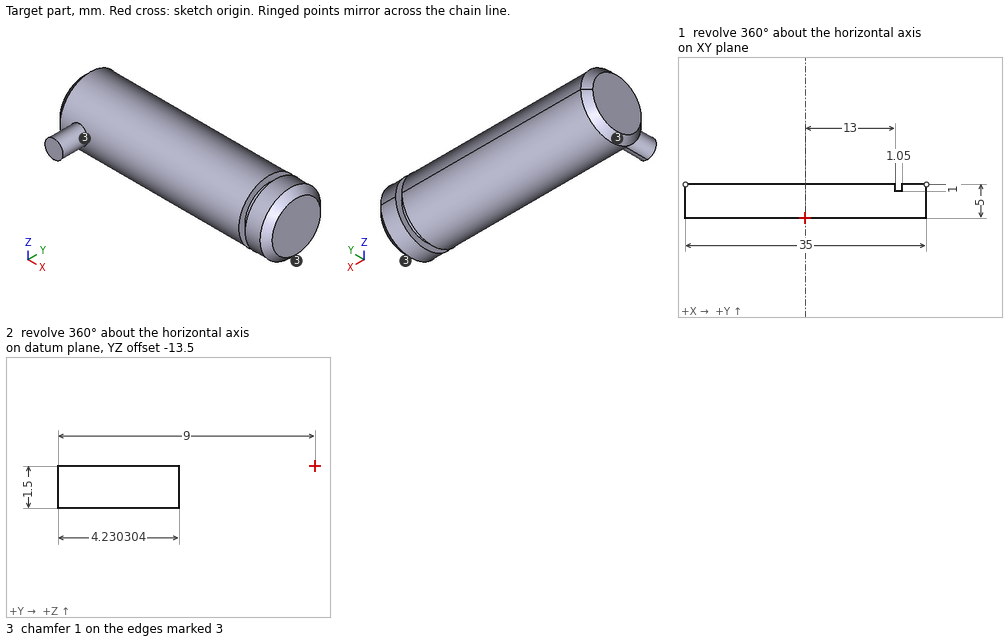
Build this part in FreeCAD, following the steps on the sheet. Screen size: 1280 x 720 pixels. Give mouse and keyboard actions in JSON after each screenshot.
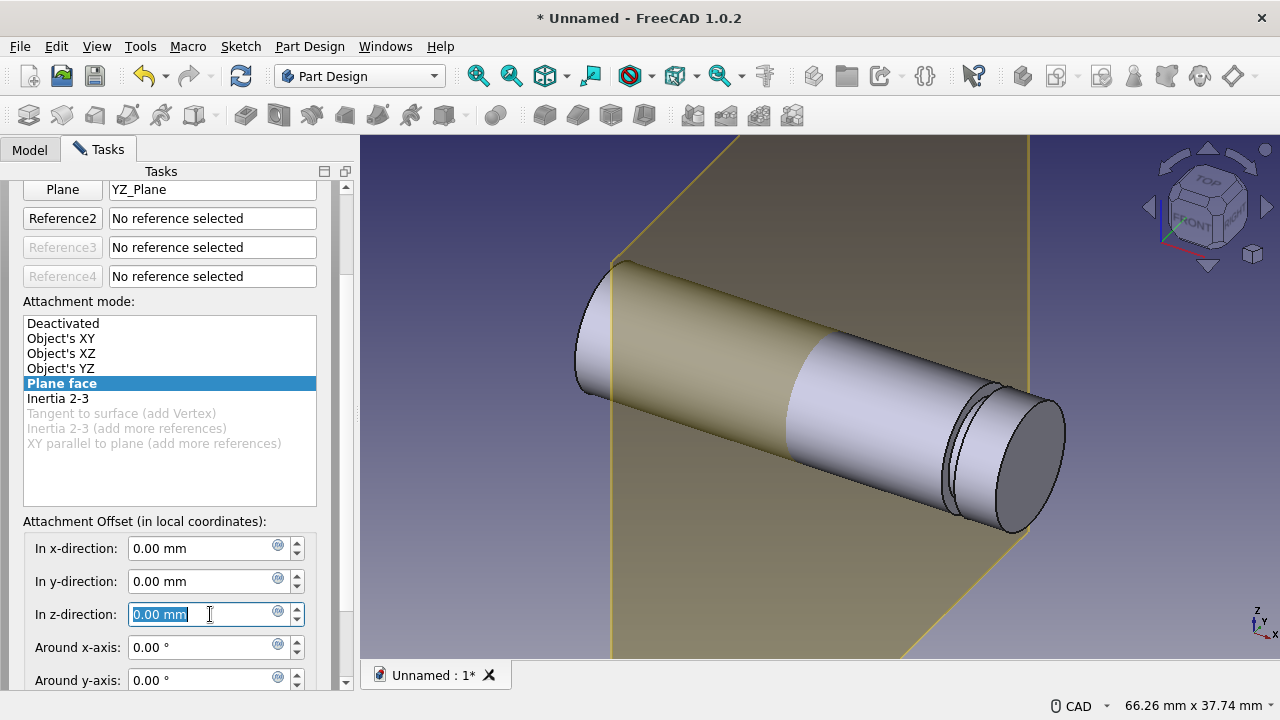
{"action": "type", "text": "-13.5"}
{"action": "key", "text": "Tab"}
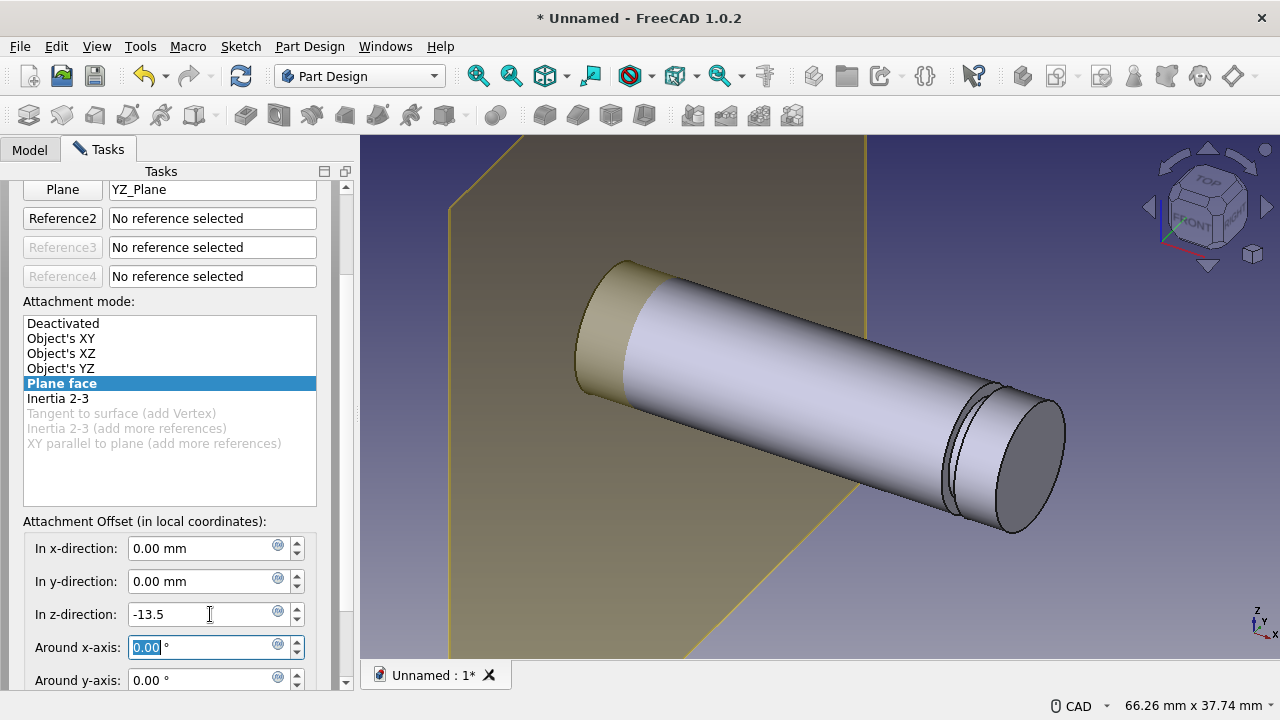
{"action": "scroll", "coordinate": [346, 436], "scroll_direction": "up", "scroll_amount": 3}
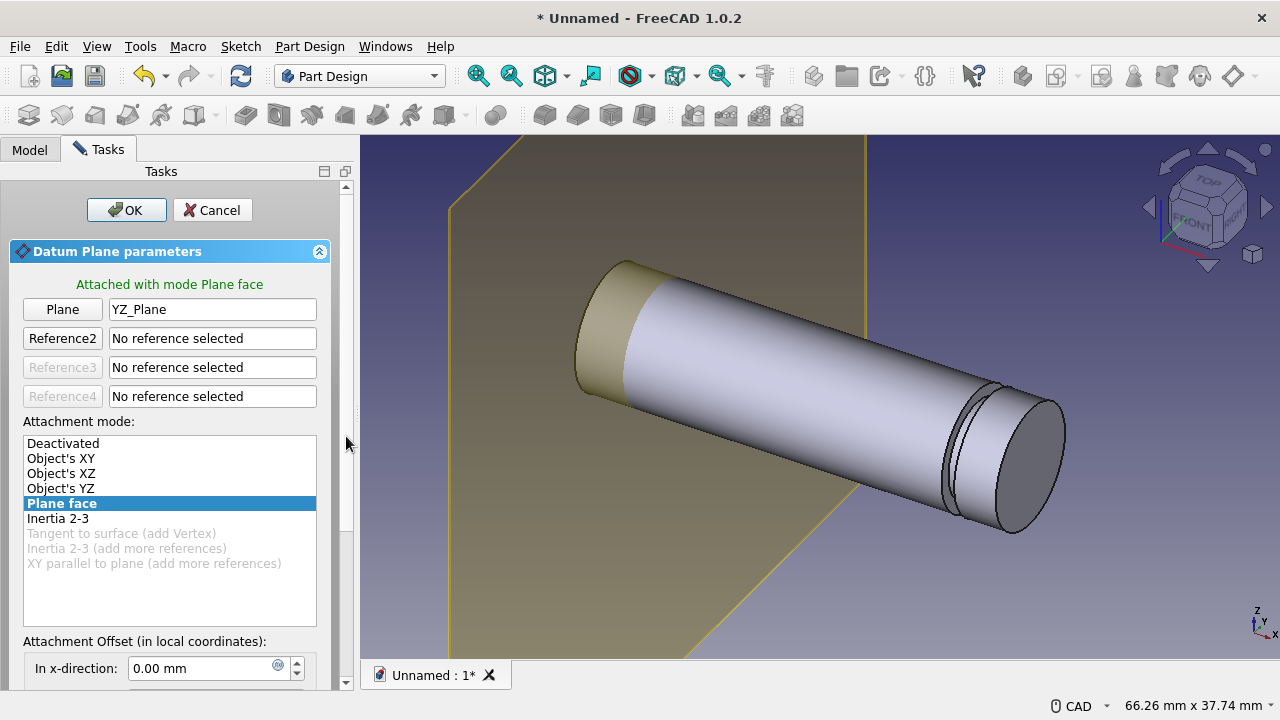
{"action": "left_click", "coordinate": [127, 210]}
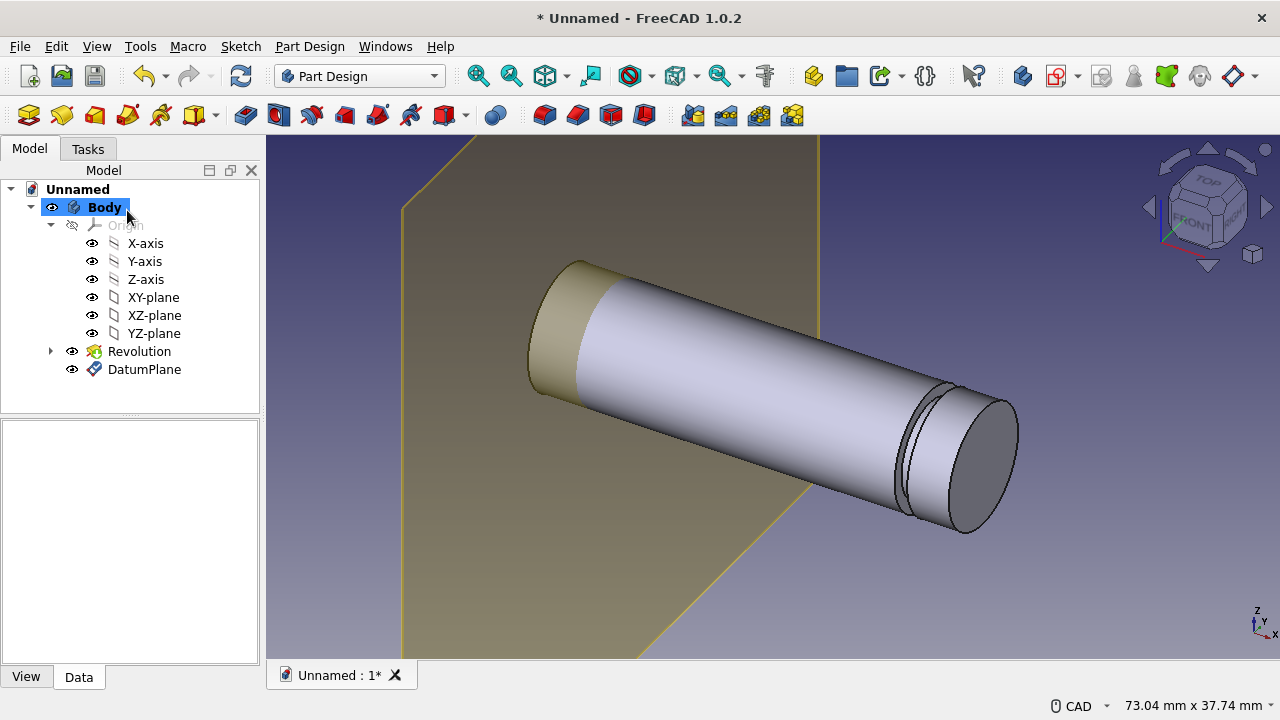
{"action": "left_click", "coordinate": [117, 369]}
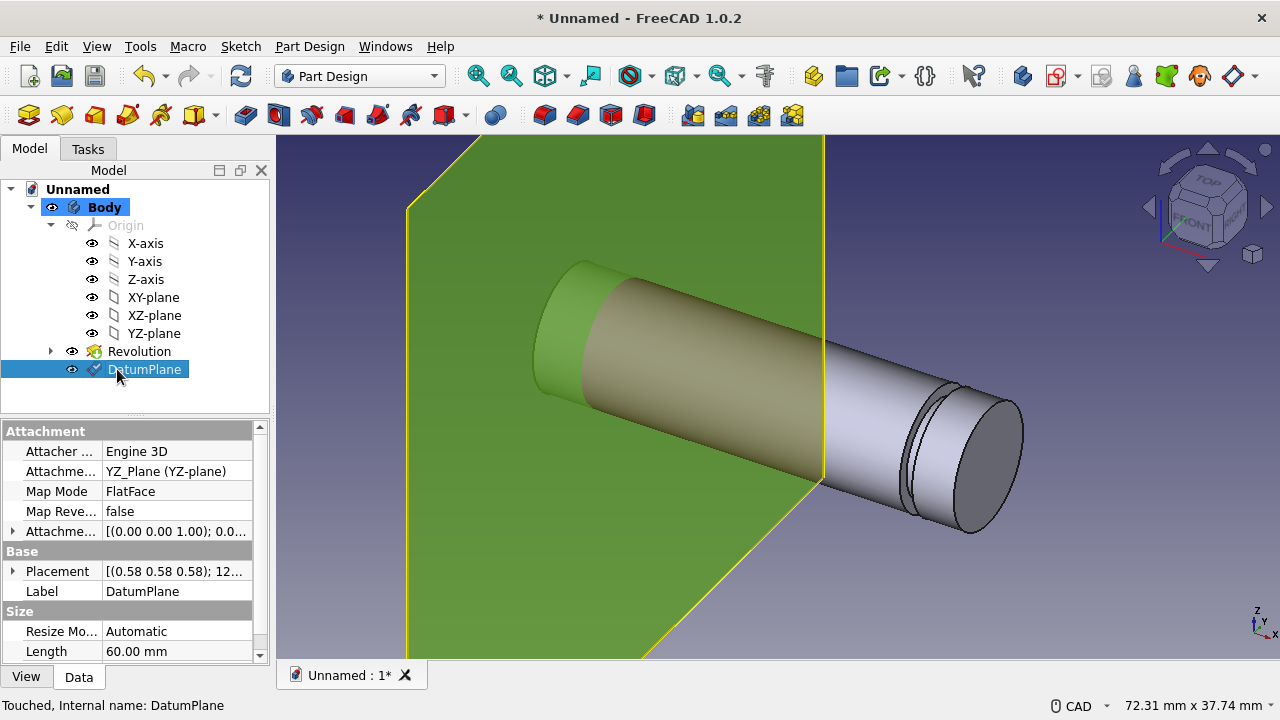
{"action": "left_click", "coordinate": [1056, 76]}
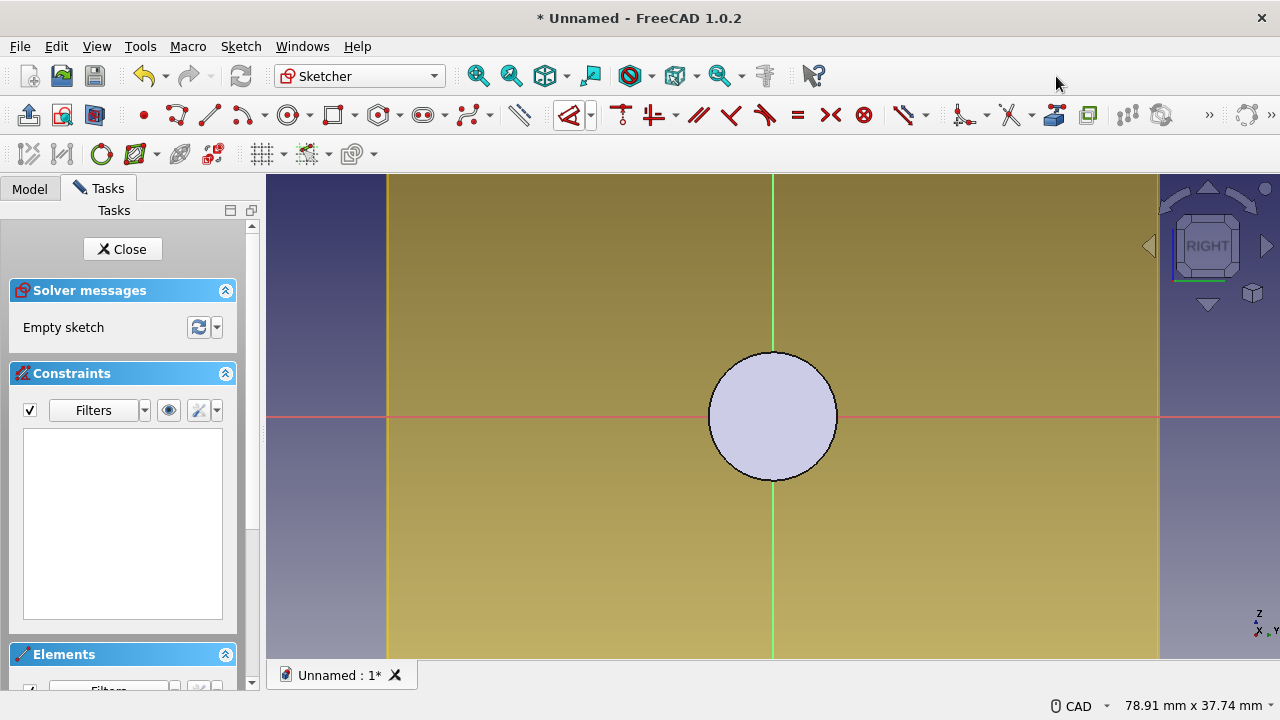
{"action": "left_click", "coordinate": [95, 116]}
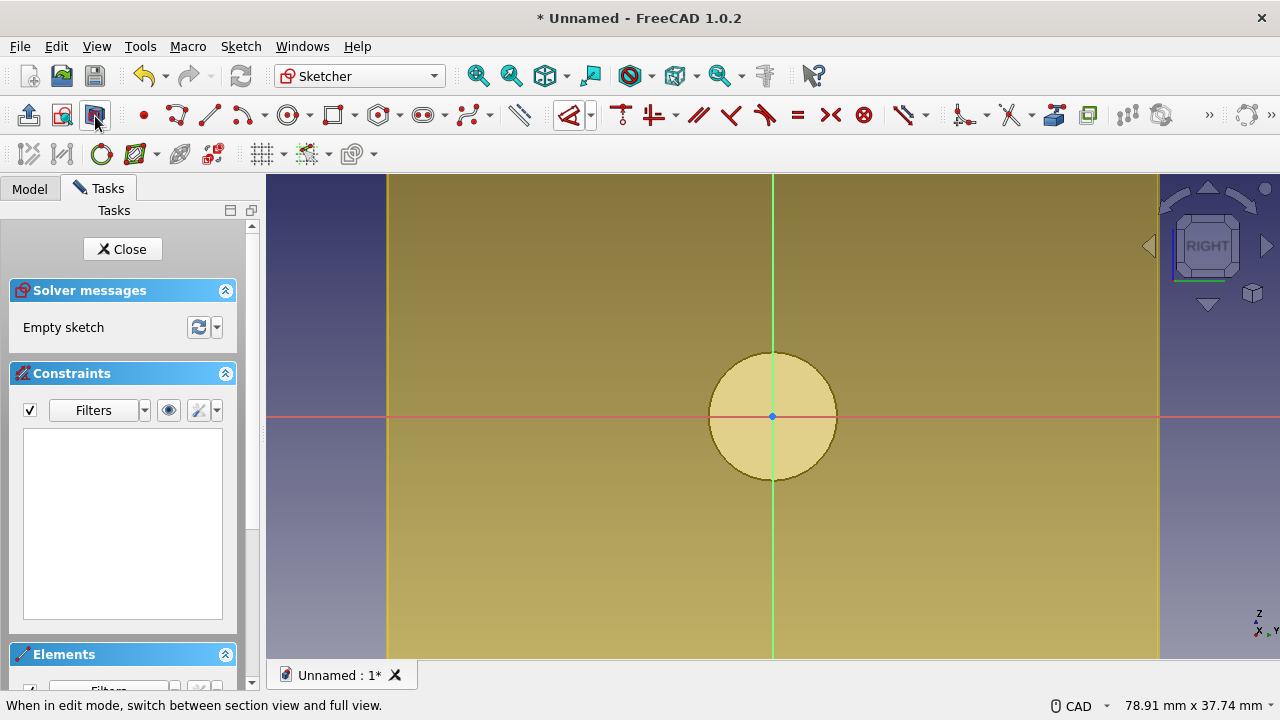
{"action": "scroll", "coordinate": [718, 429], "scroll_direction": "up", "scroll_amount": 8}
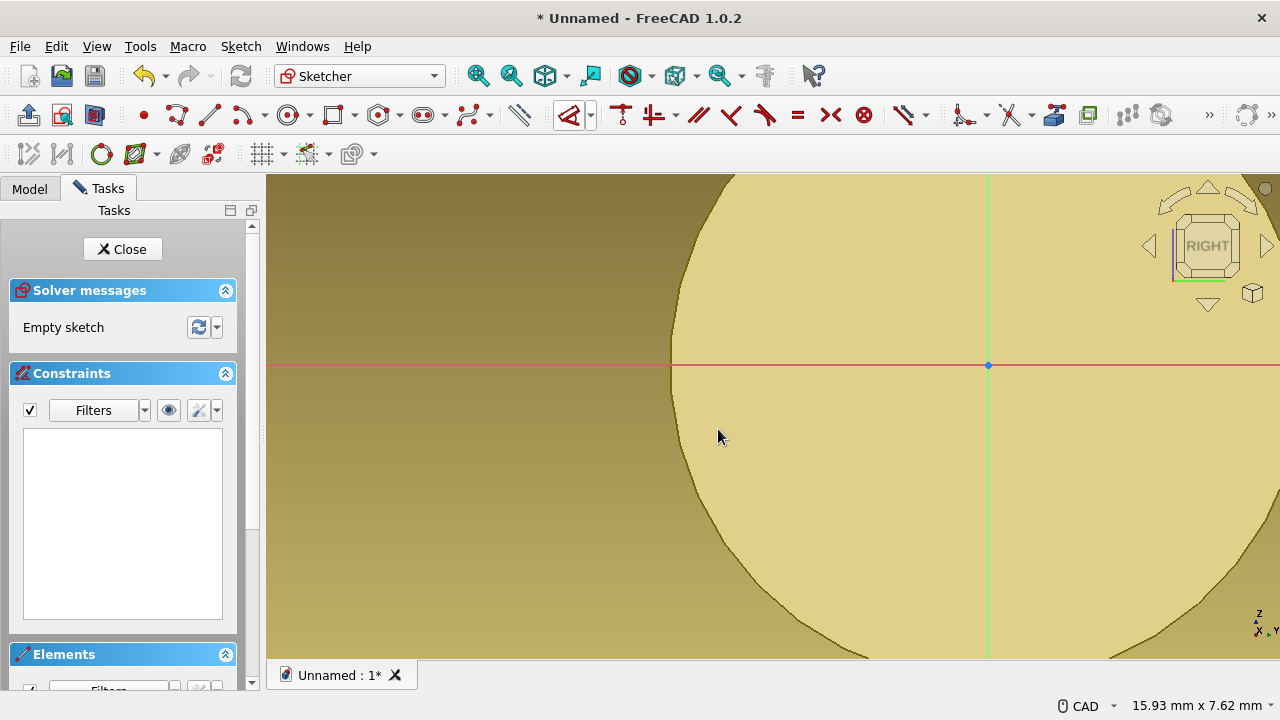
{"action": "left_click", "coordinate": [332, 116]}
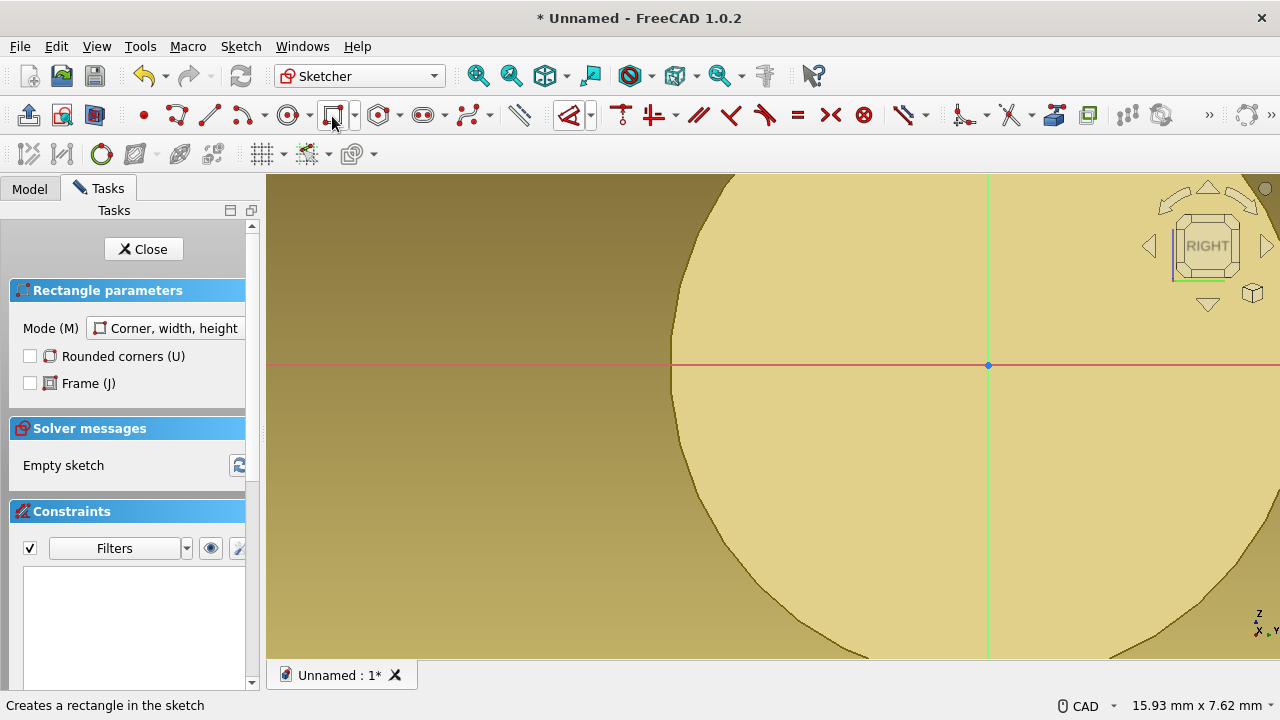
{"action": "left_click", "coordinate": [415, 365]}
{"action": "mouse_move", "coordinate": [684, 460]}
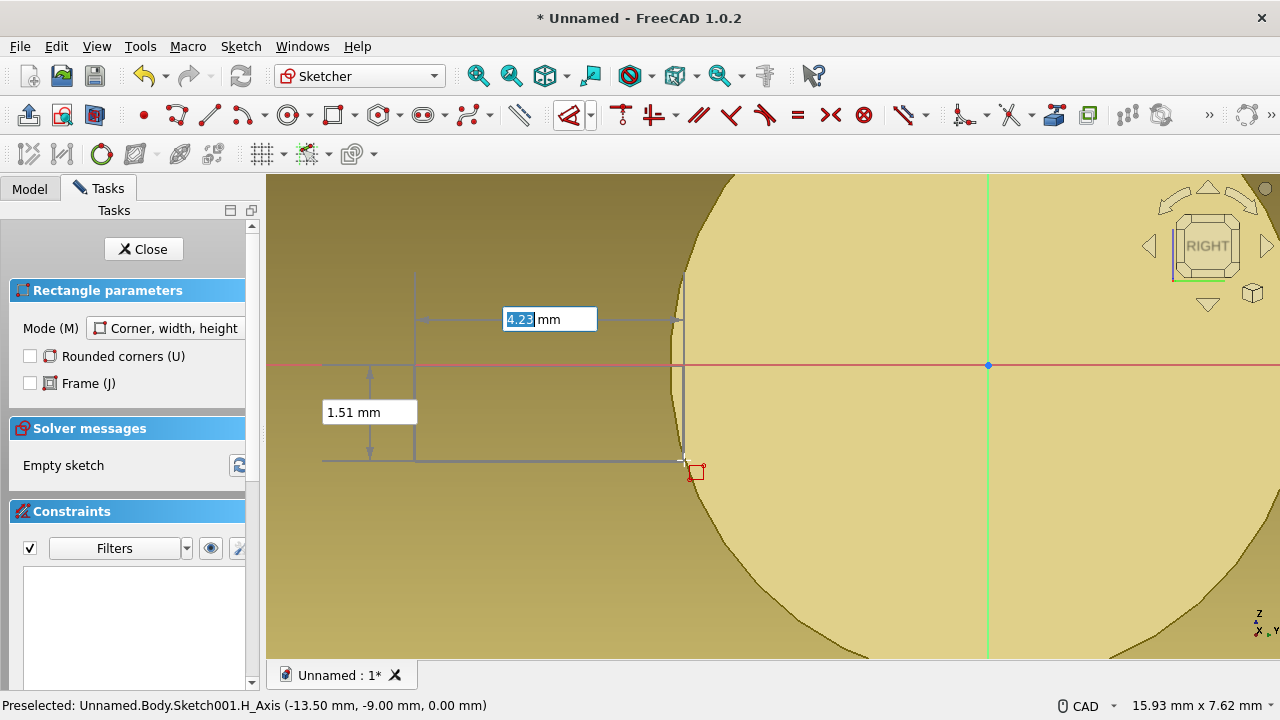
{"action": "type", "text": "4.230304"}
{"action": "key", "text": "Tab"}
{"action": "type", "text": "1.5"}
{"action": "key", "text": "Return"}
{"action": "key", "text": "Escape"}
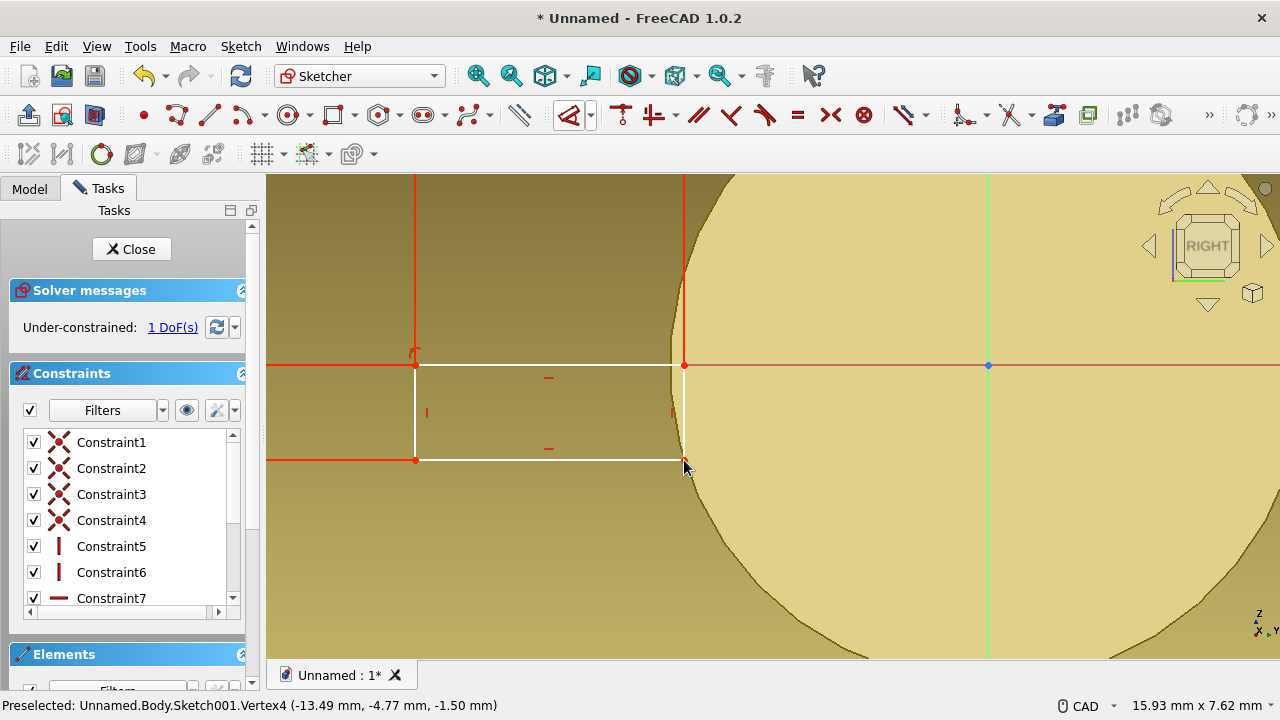
{"action": "left_click", "coordinate": [415, 365]}